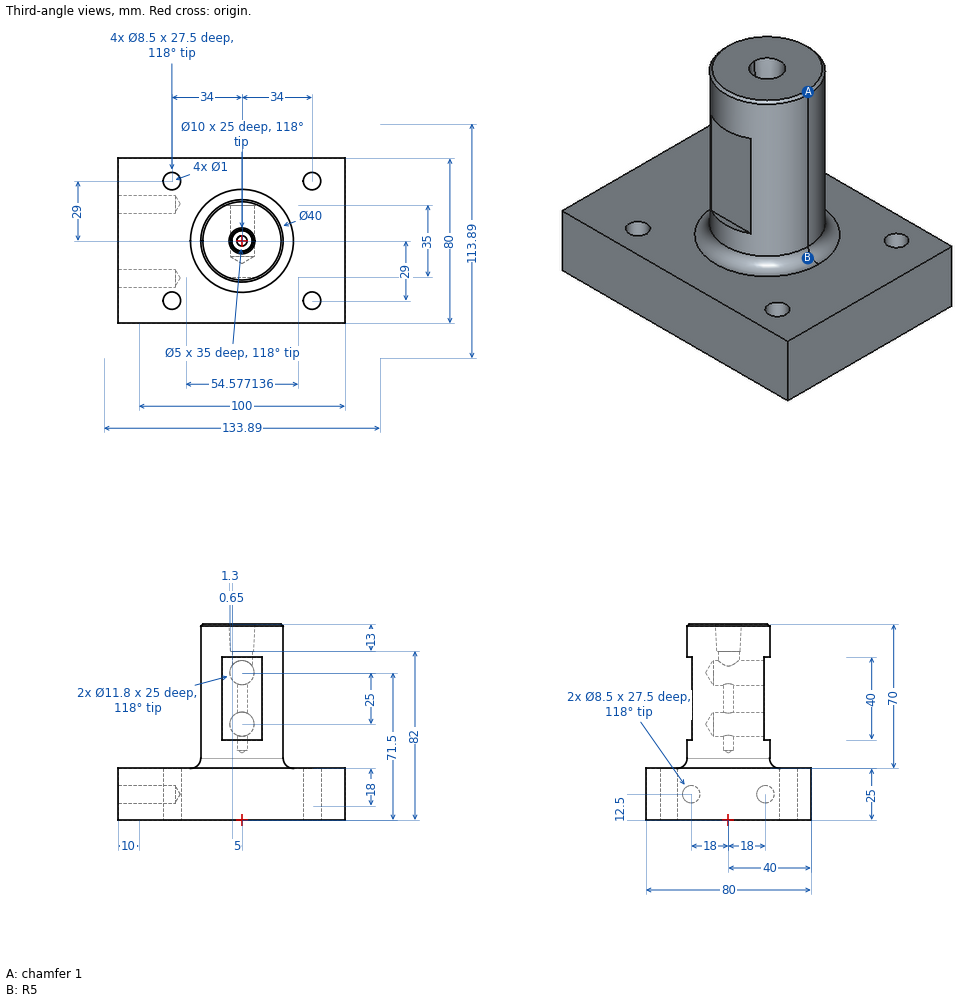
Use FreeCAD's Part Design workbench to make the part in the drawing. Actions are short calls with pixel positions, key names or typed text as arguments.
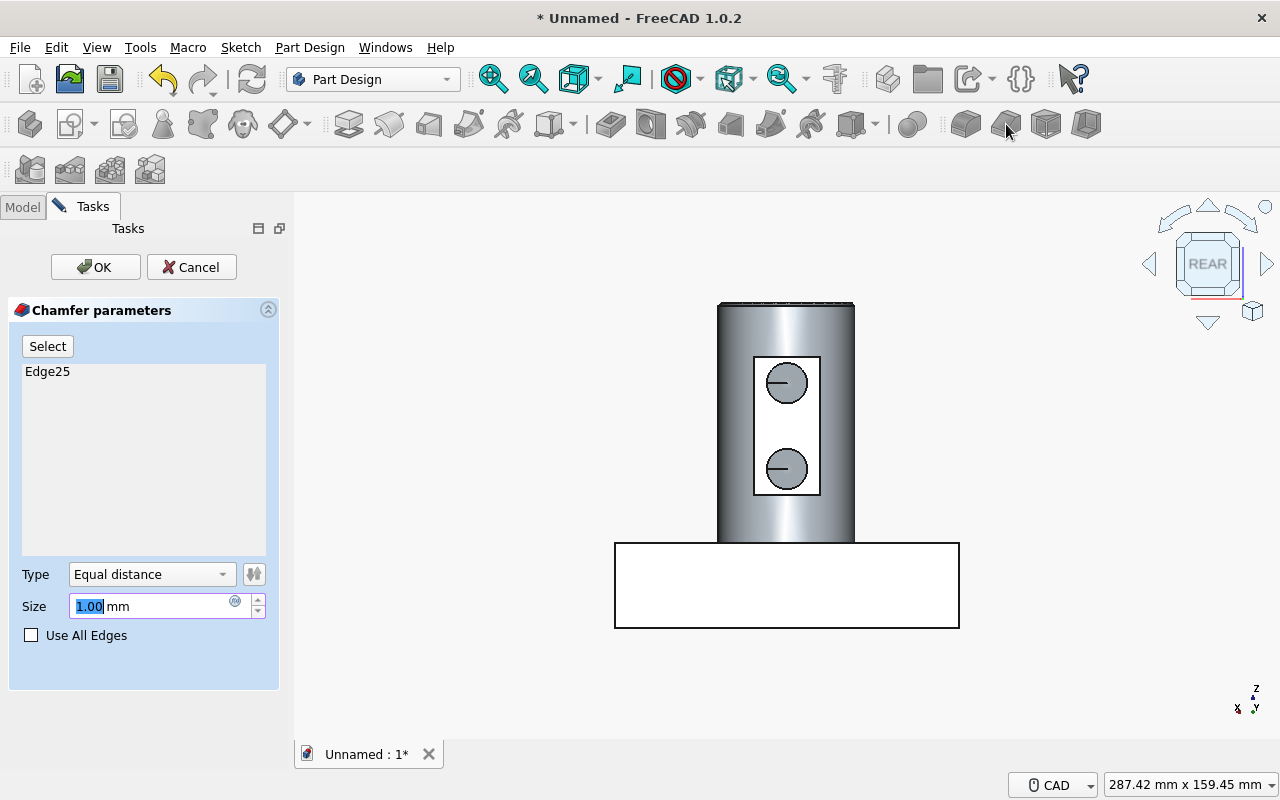
text(1)
key(Tab)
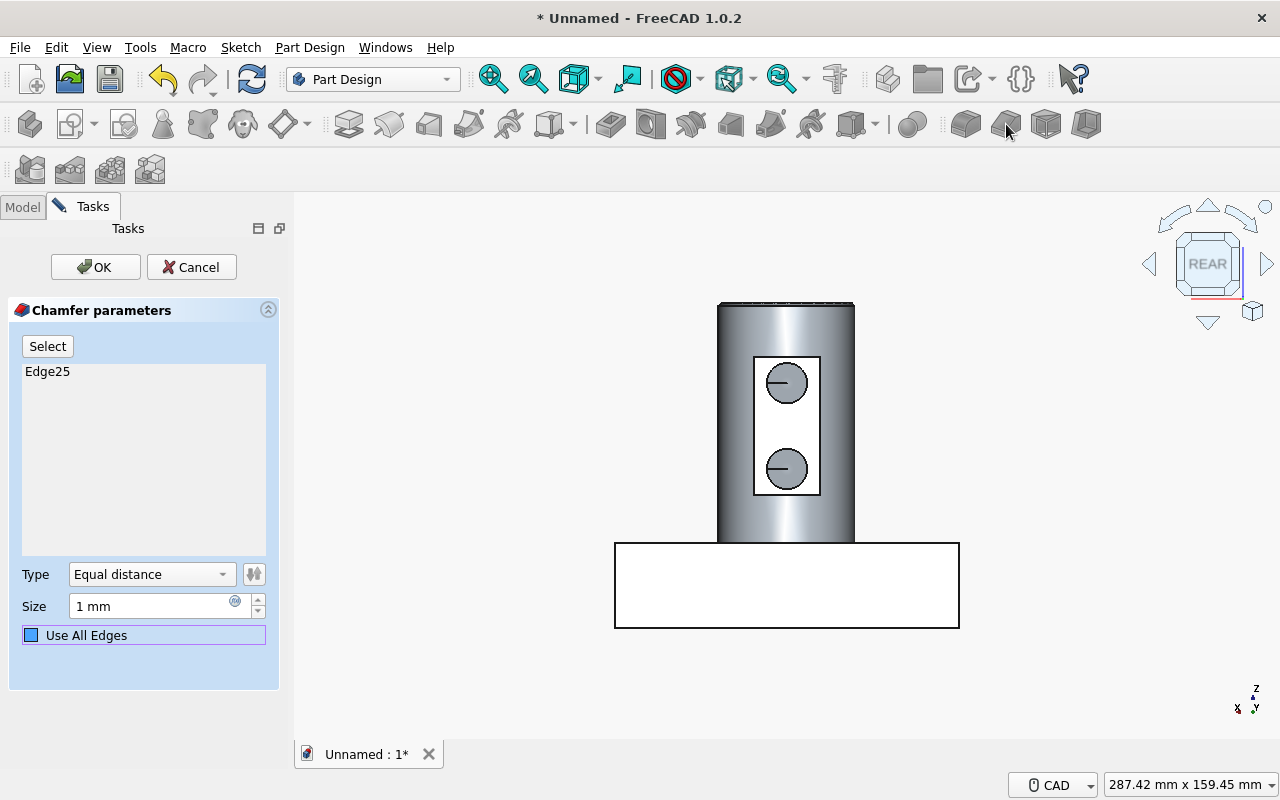
click(96, 267)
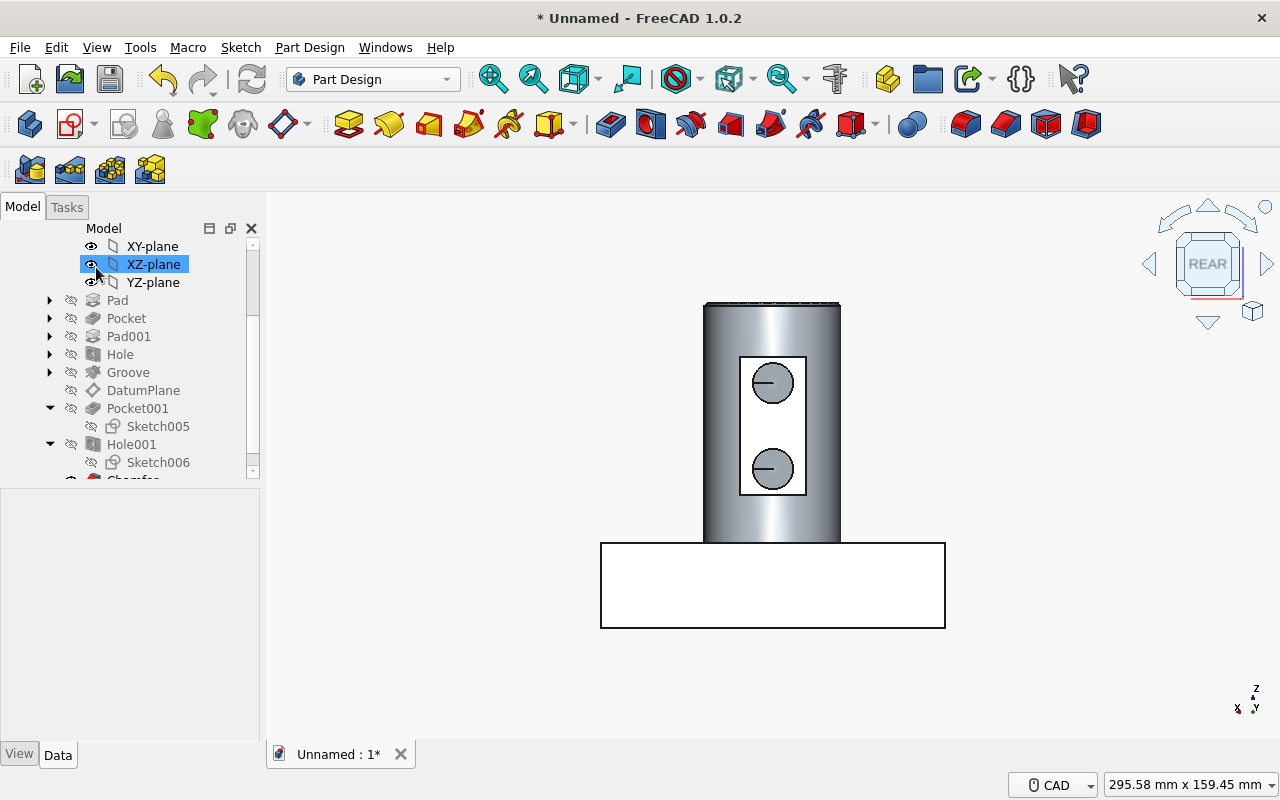
key(0)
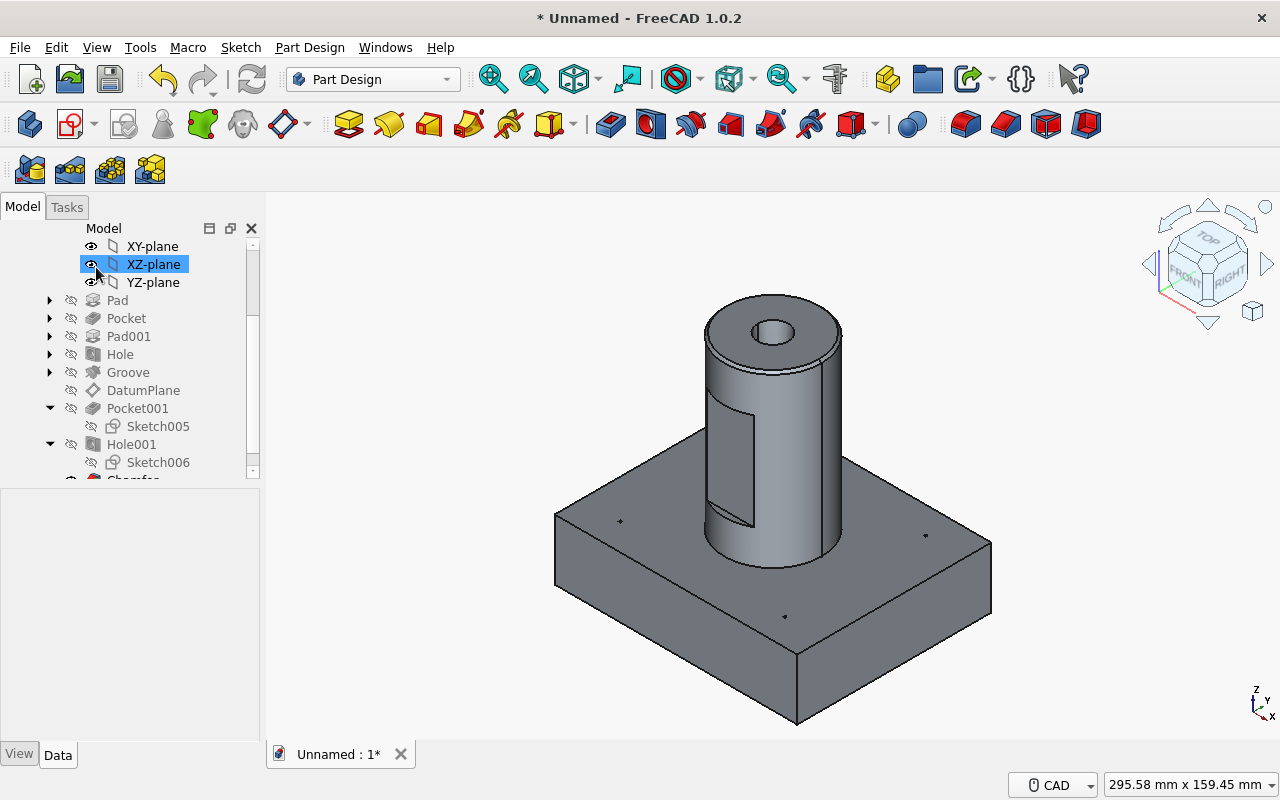
click(676, 504)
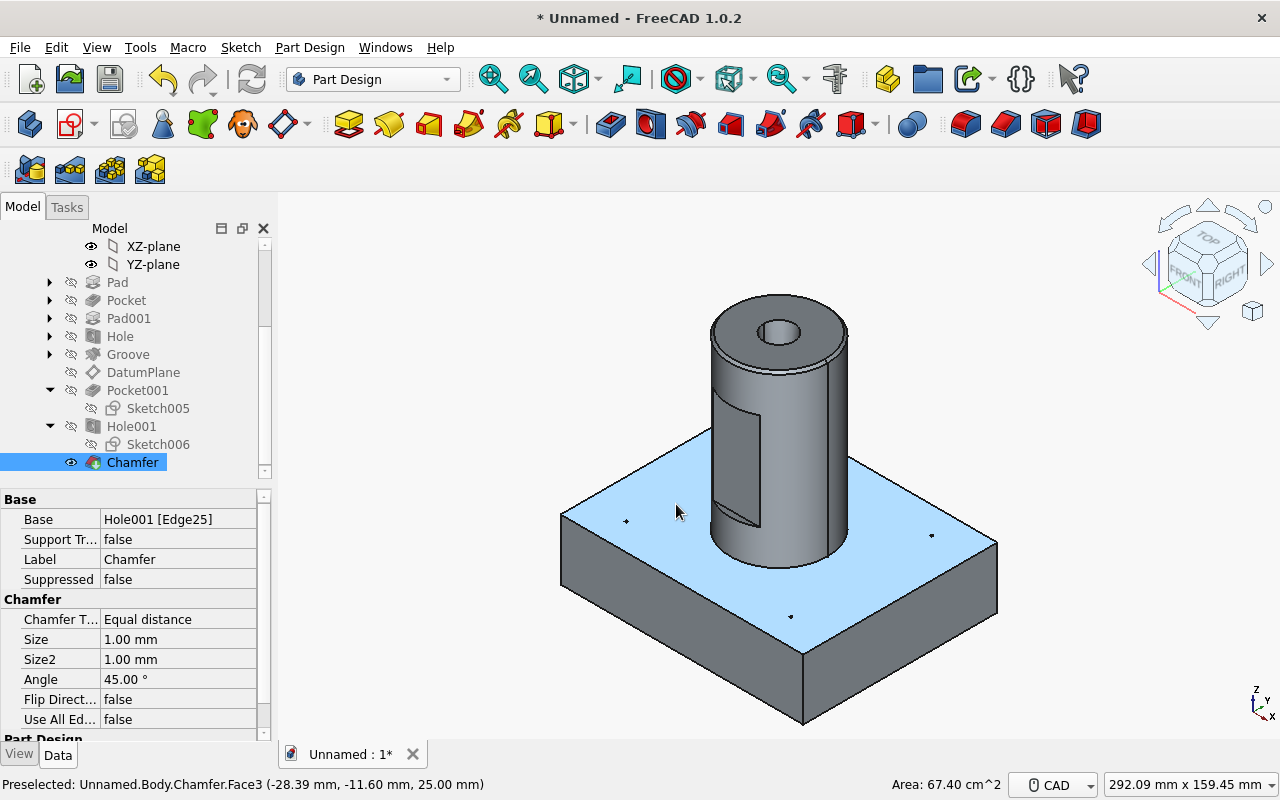
click(70, 124)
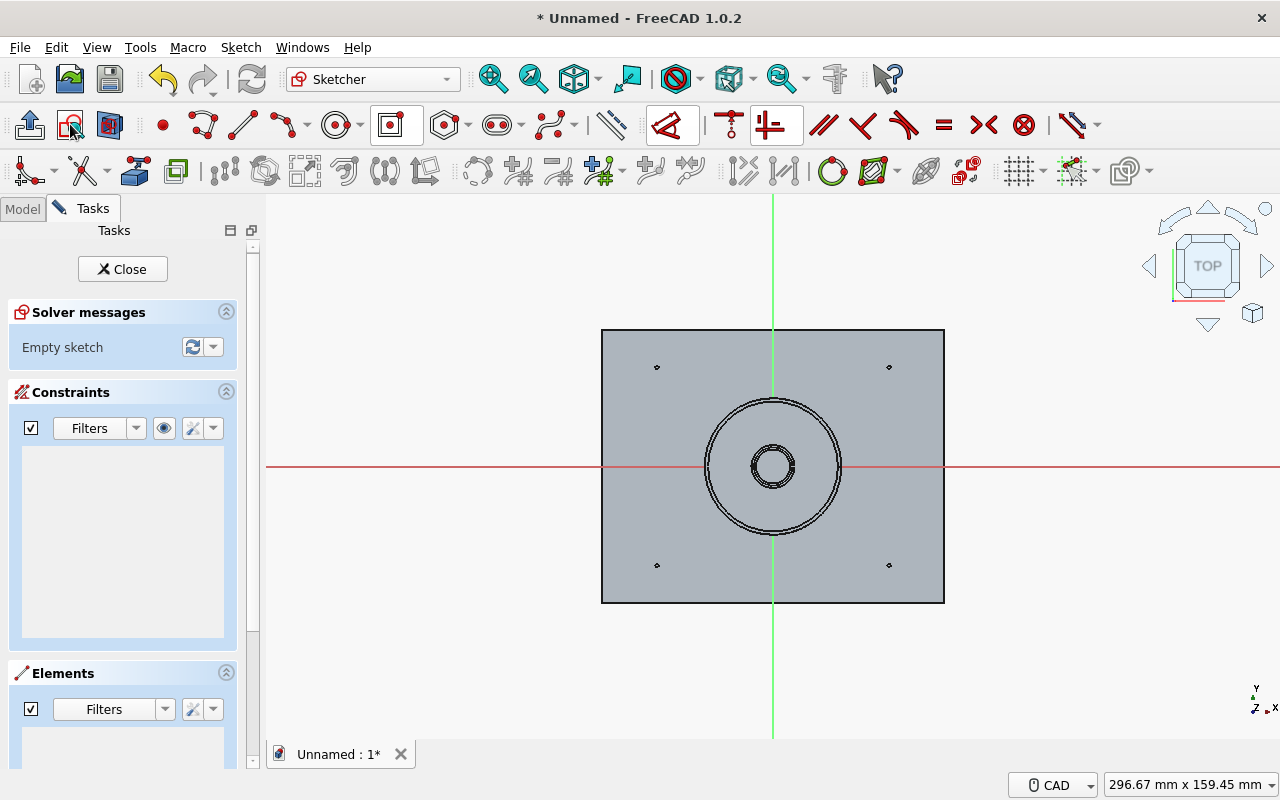
click(110, 126)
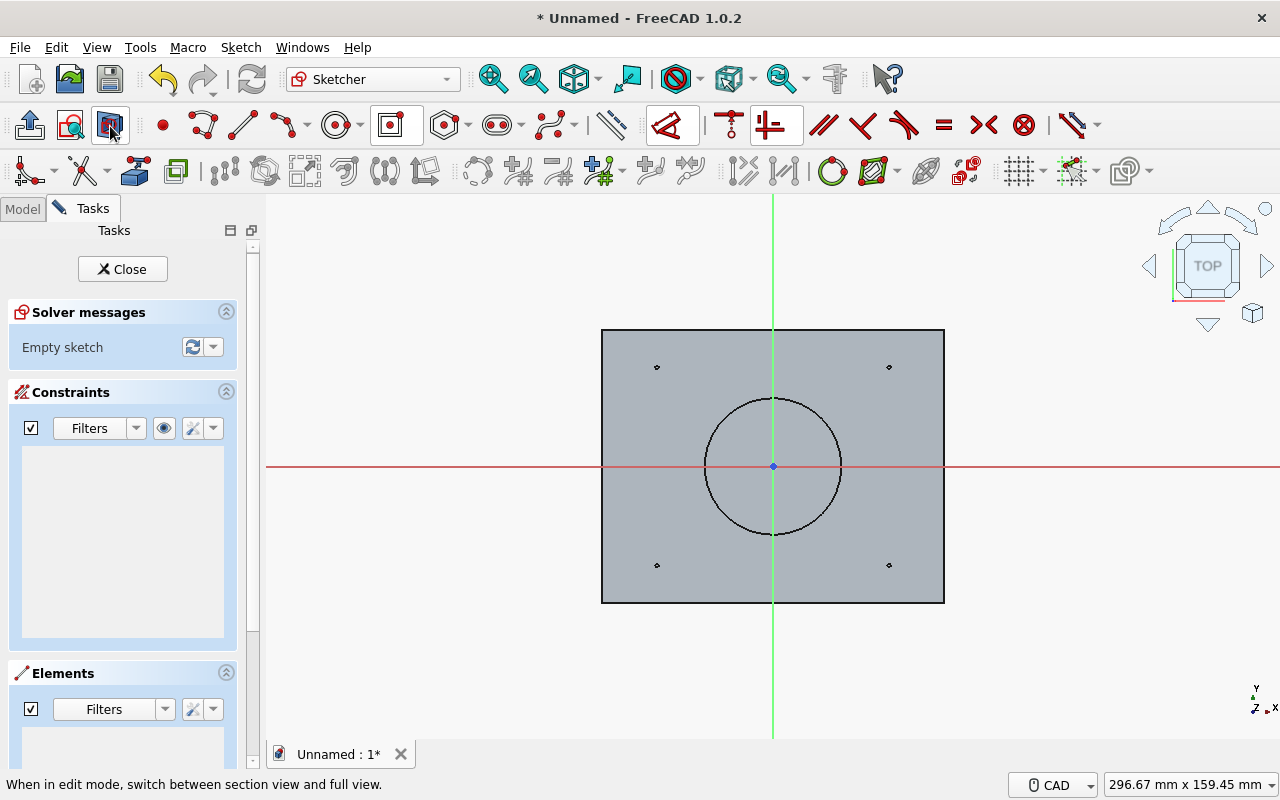
scroll(912, 467, up, 2)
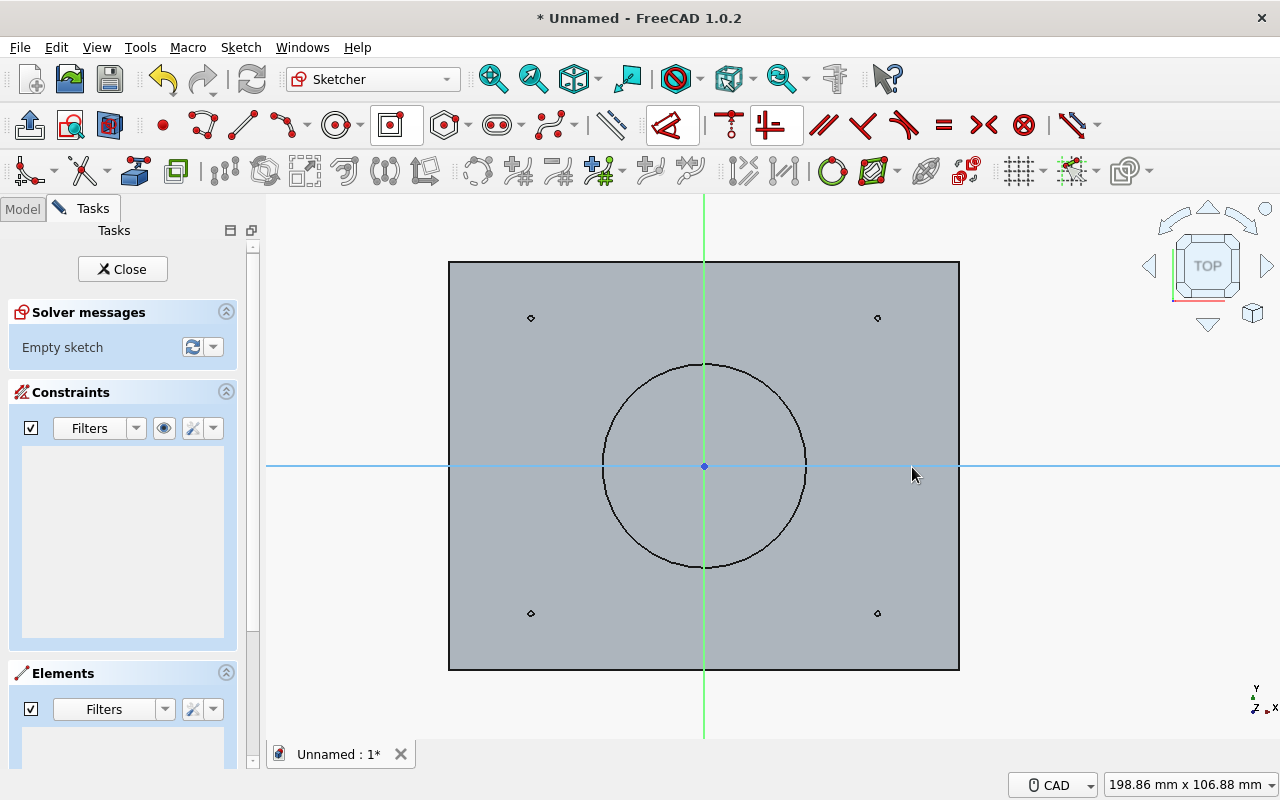
key(g)
key(c)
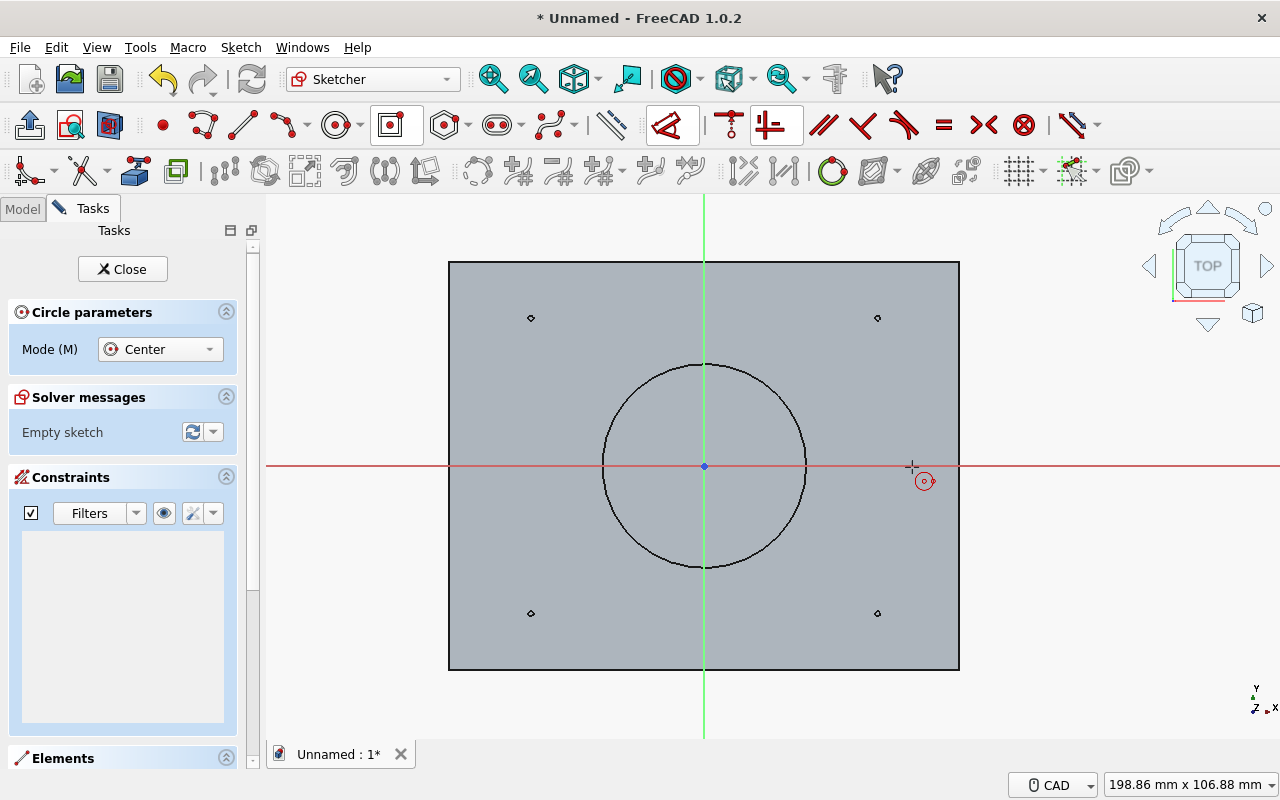
click(531, 318)
click(546, 303)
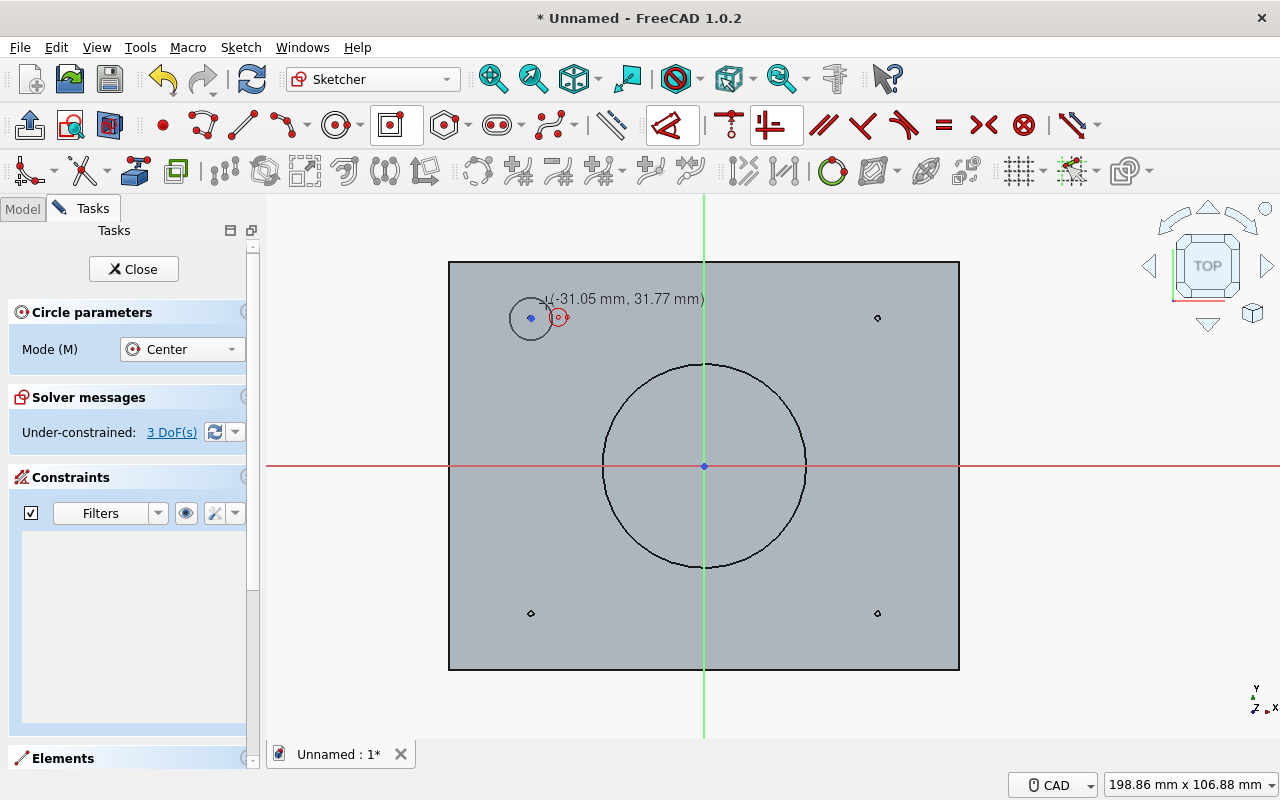
click(878, 318)
click(893, 303)